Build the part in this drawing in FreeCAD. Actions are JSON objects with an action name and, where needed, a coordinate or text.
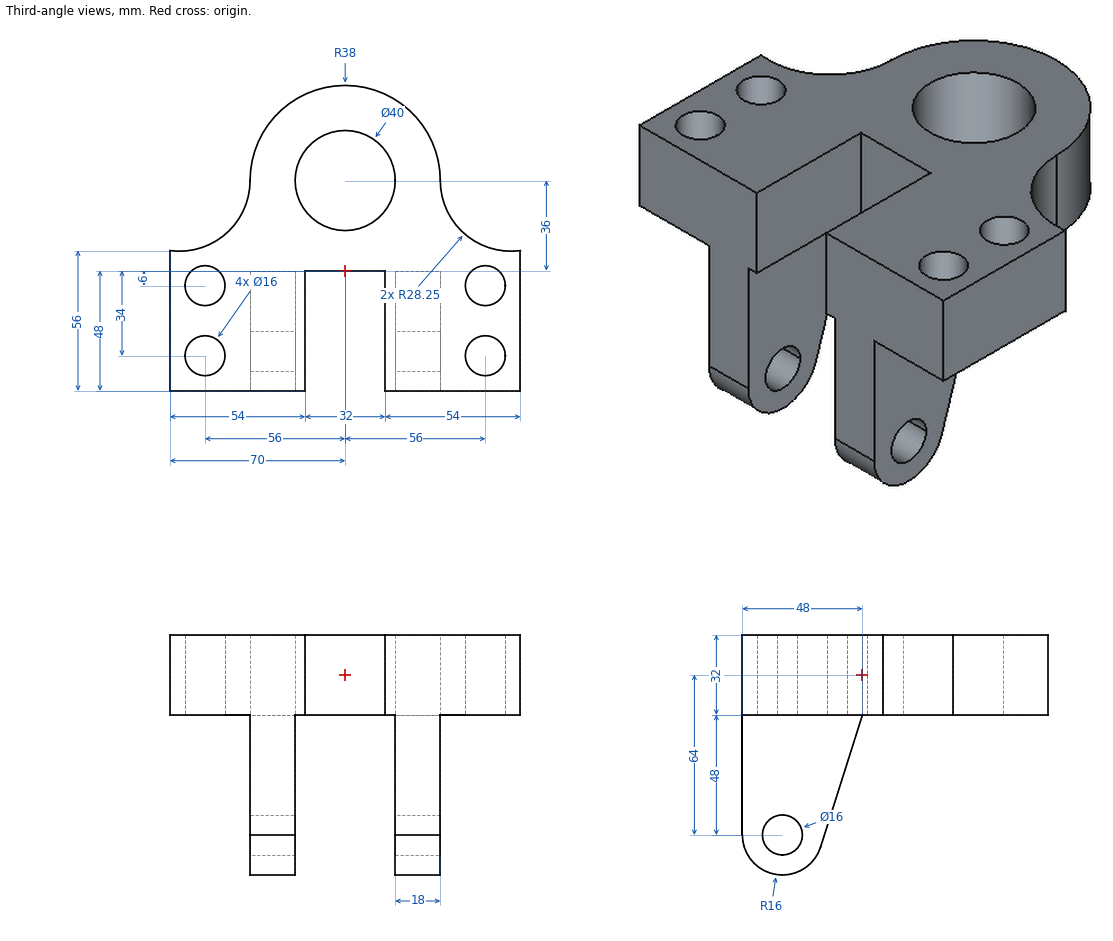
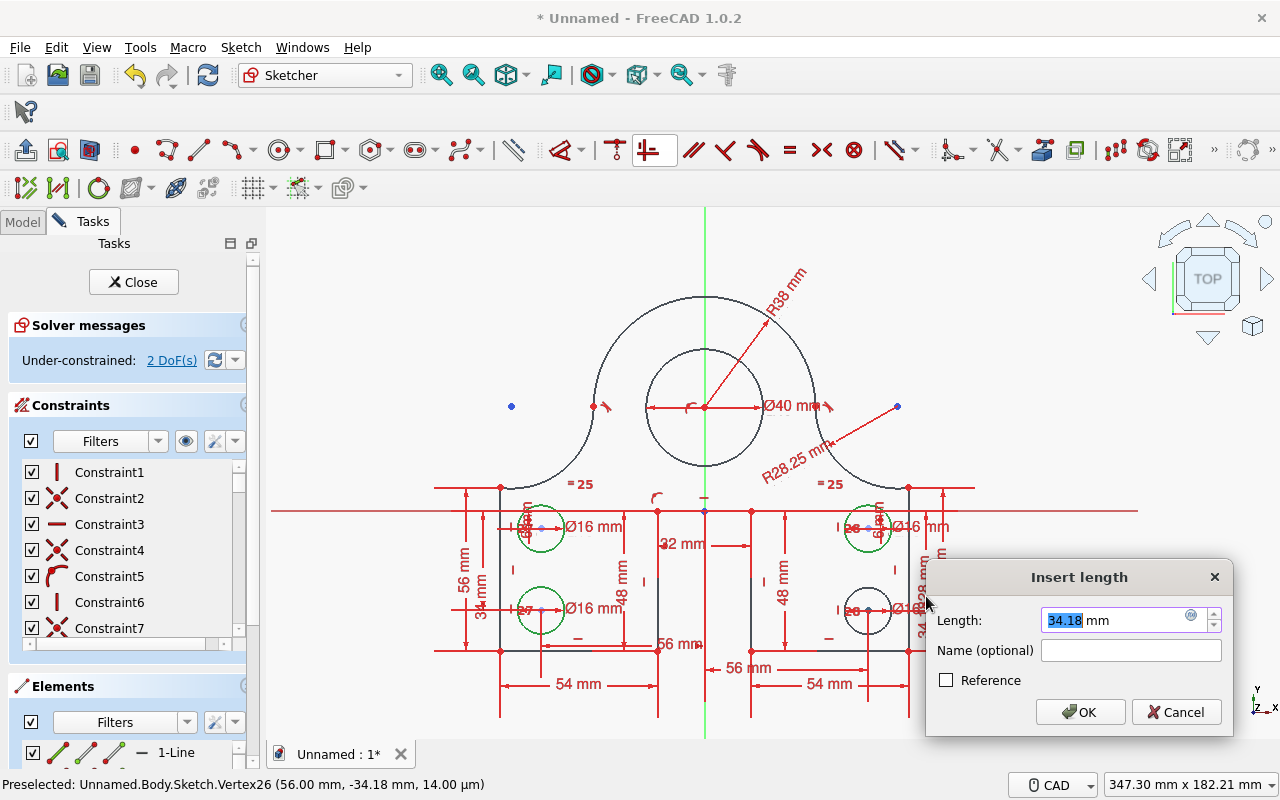
{"action": "type", "text": "34"}
{"action": "key", "text": "Return"}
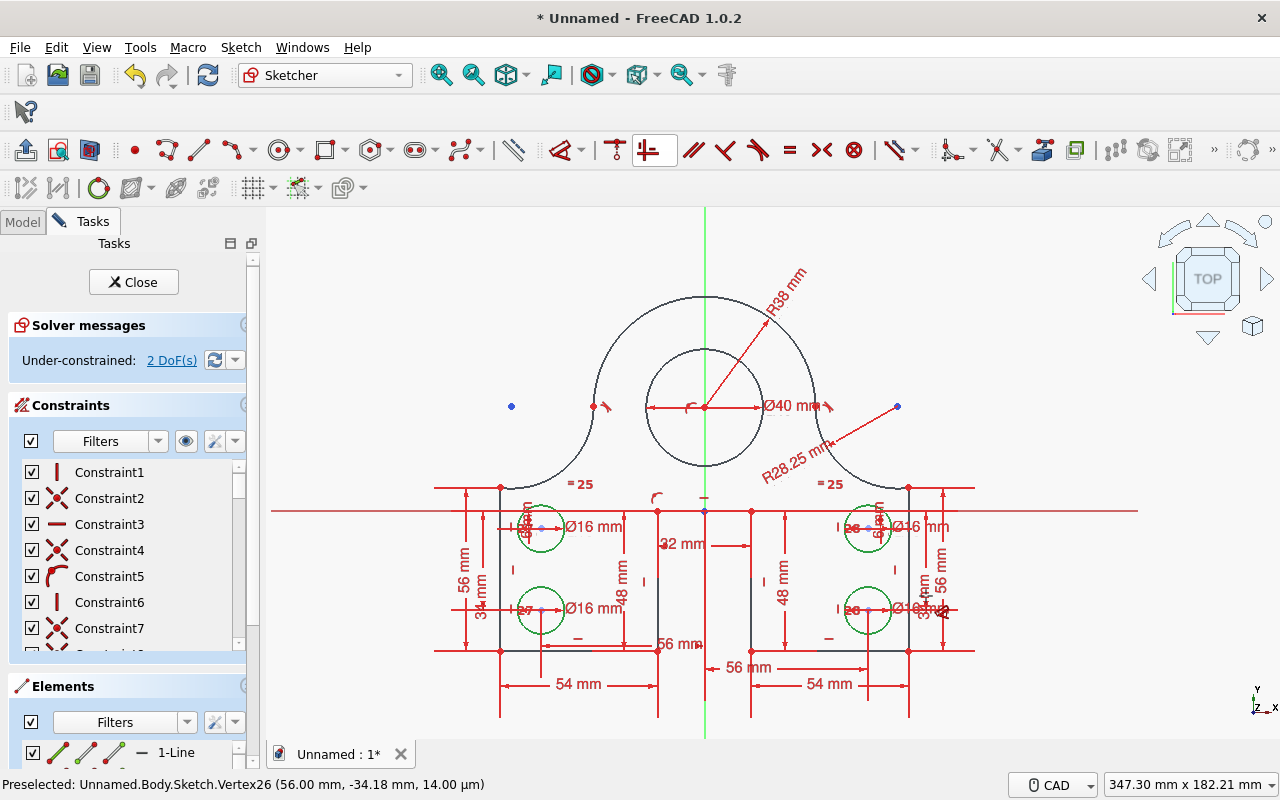
{"action": "left_click", "coordinate": [705, 408]}
{"action": "left_click", "coordinate": [739, 436]}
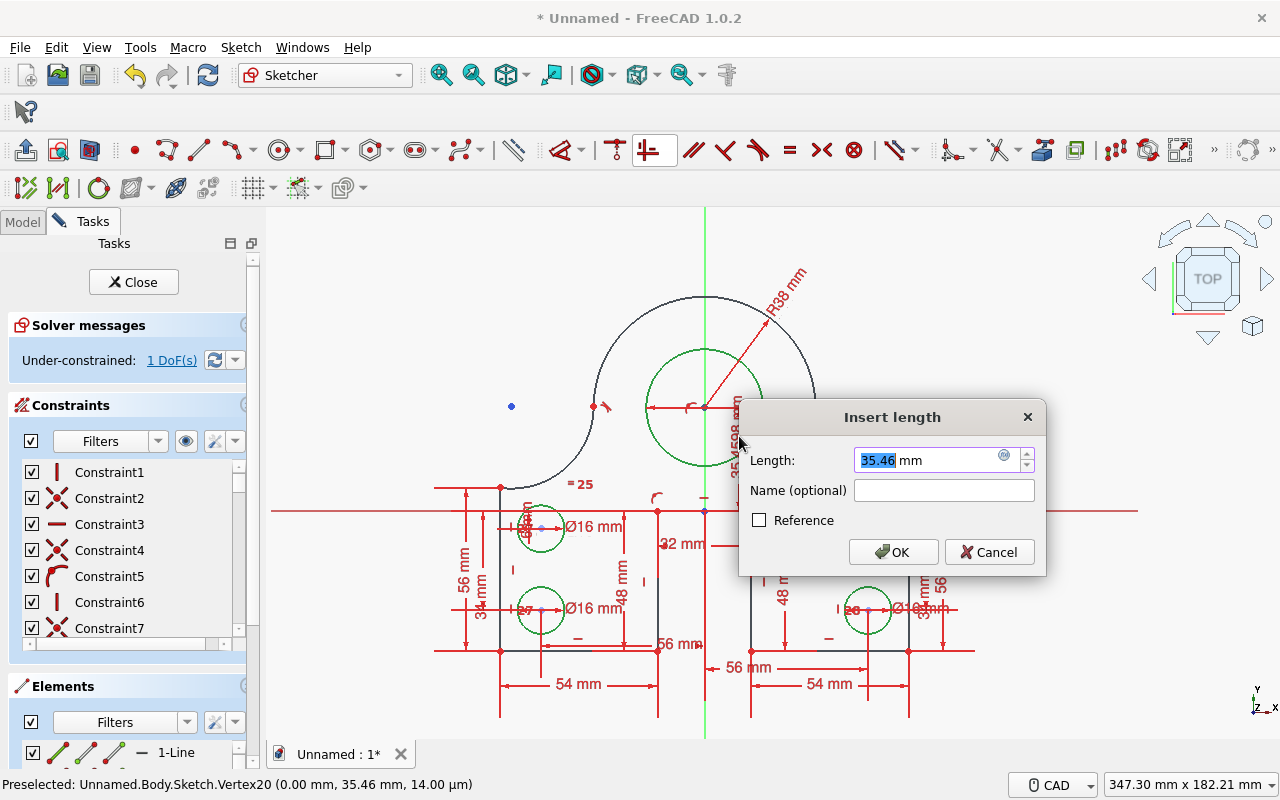
{"action": "type", "text": "36"}
{"action": "key", "text": "Return"}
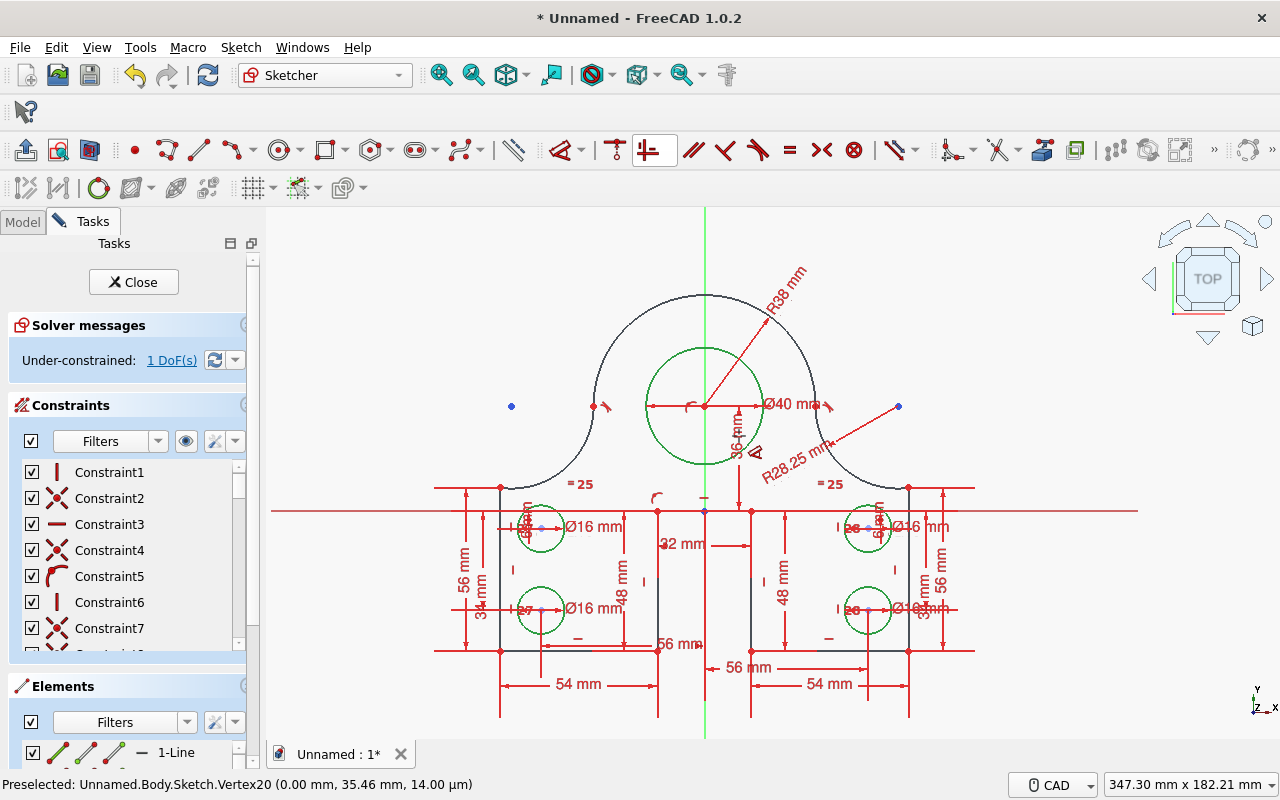
{"action": "left_click", "coordinate": [500, 488]}
{"action": "left_click", "coordinate": [602, 545]}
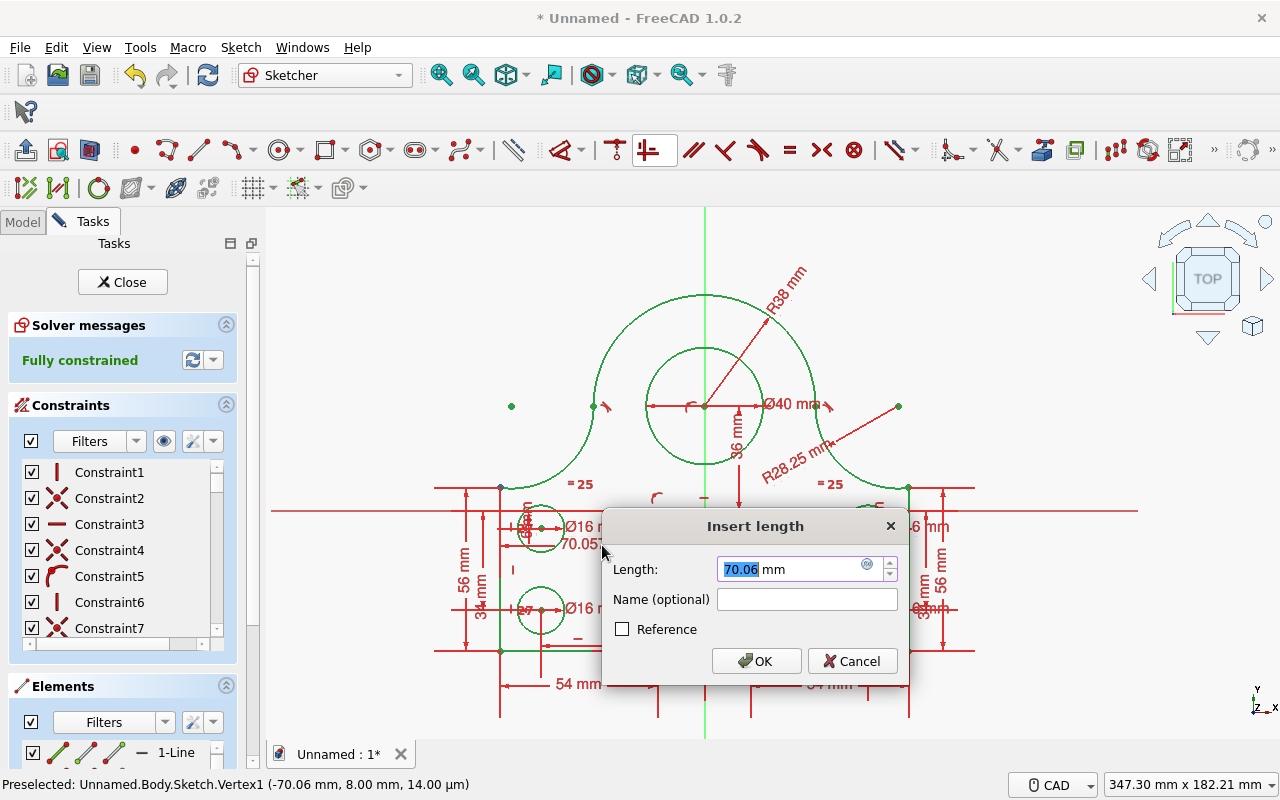
{"action": "type", "text": "70"}
{"action": "key", "text": "Return"}
{"action": "key", "text": "Escape"}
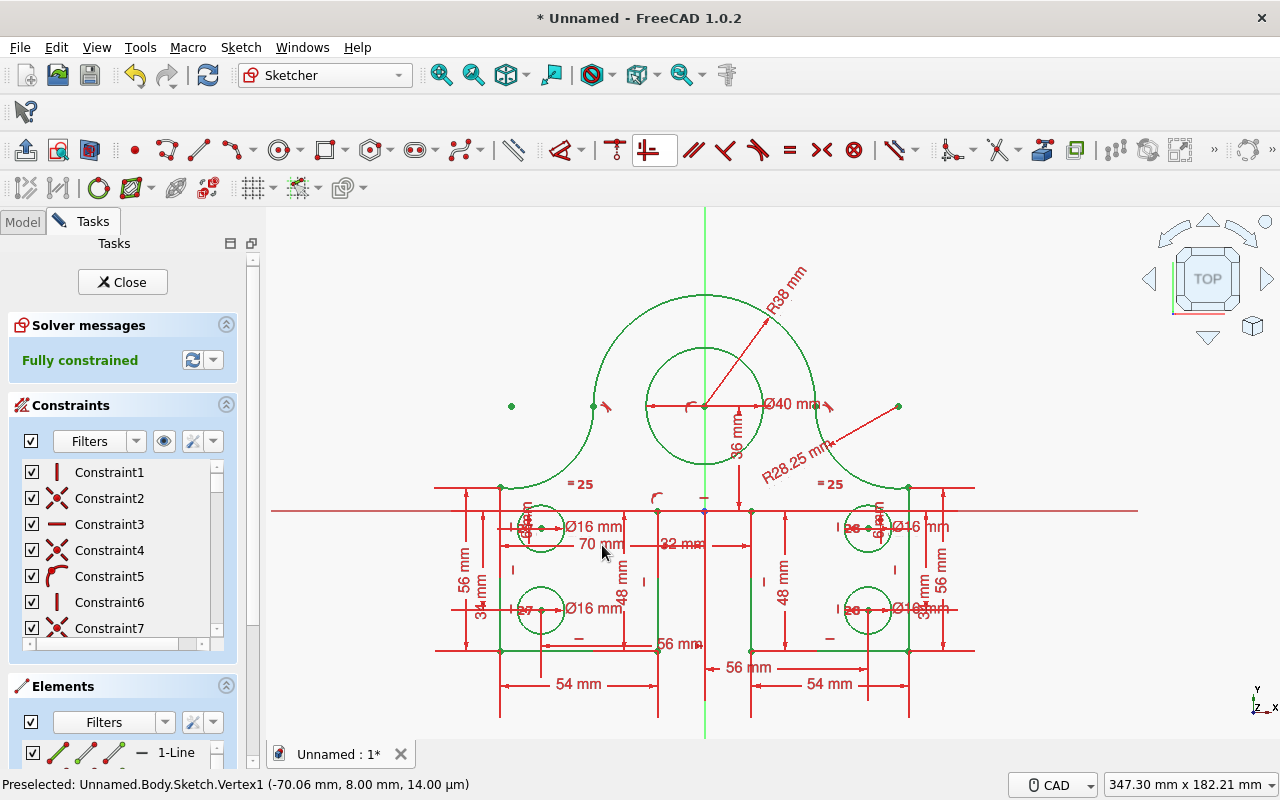
{"action": "left_click", "coordinate": [123, 282]}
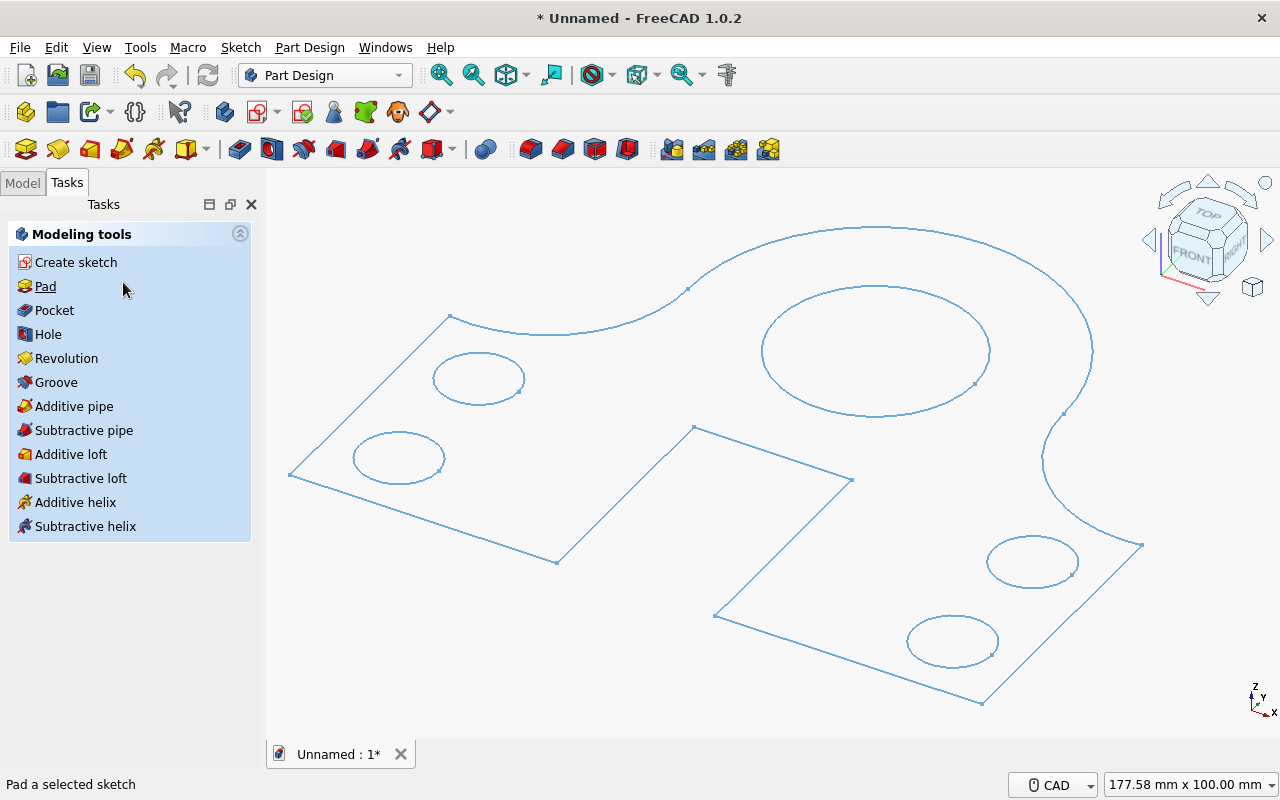
{"action": "left_click", "coordinate": [26, 150]}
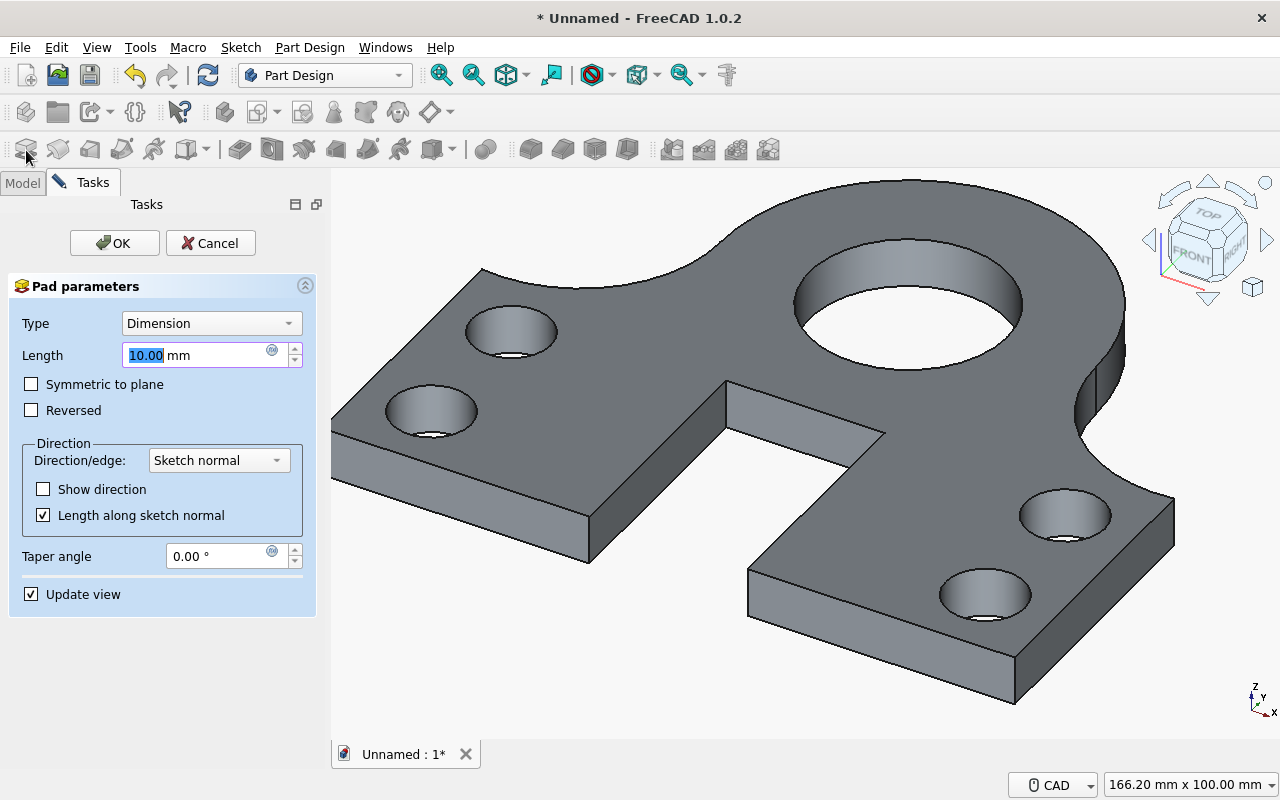
{"action": "type", "text": "32"}
{"action": "key", "text": "Tab"}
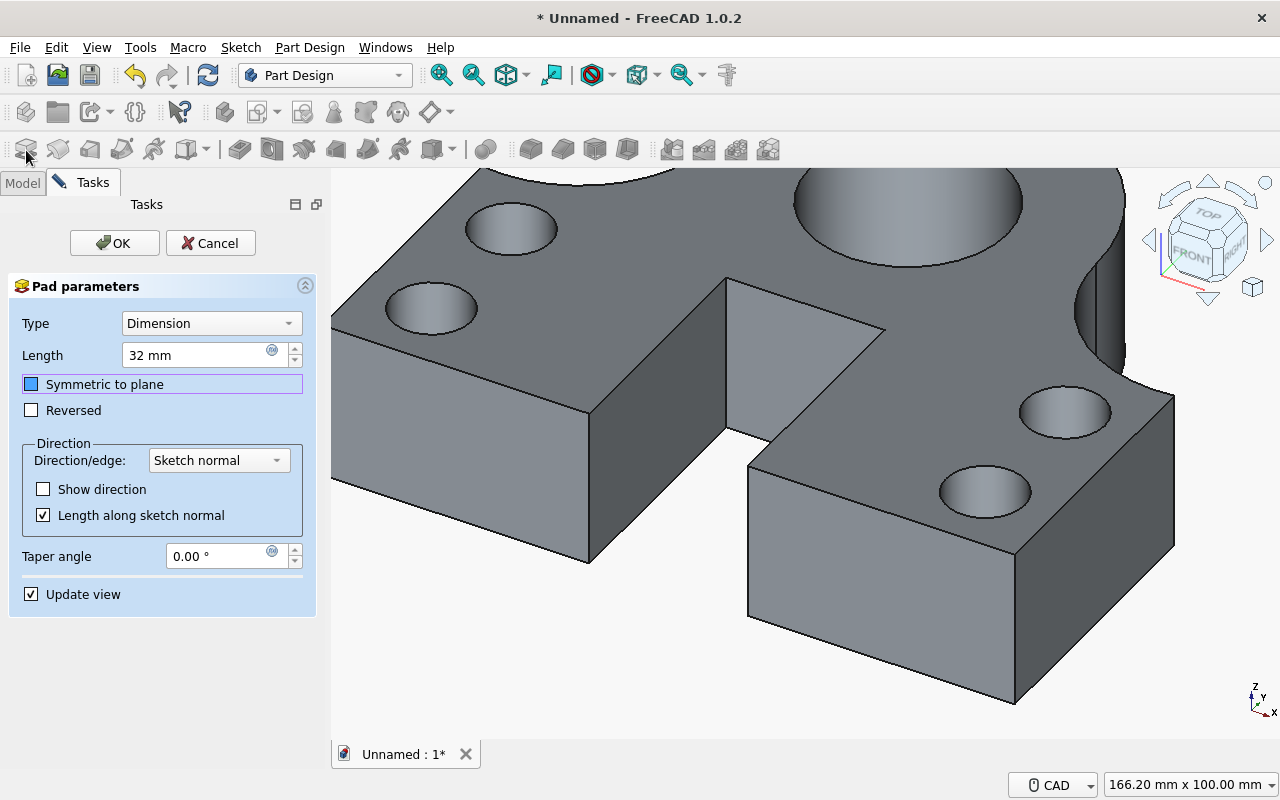
{"action": "left_click", "coordinate": [30, 384]}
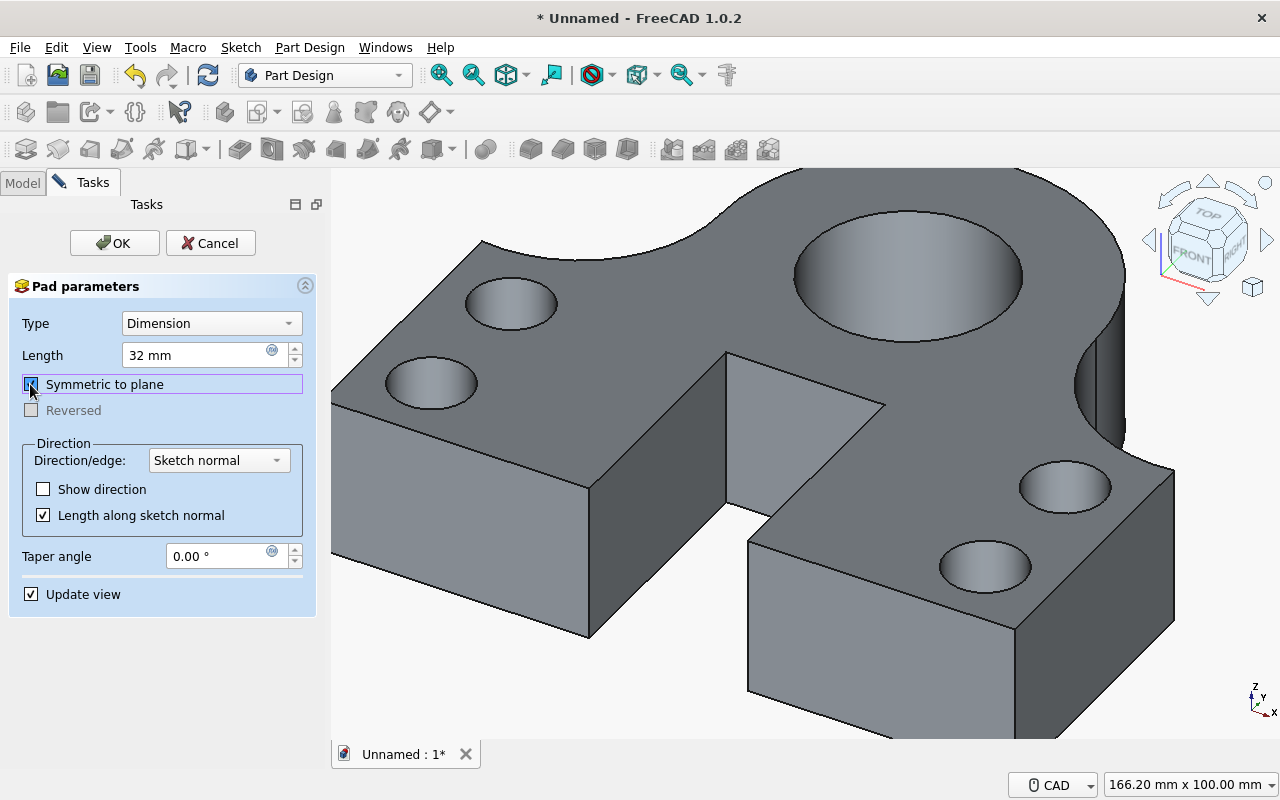
{"action": "left_click", "coordinate": [115, 243]}